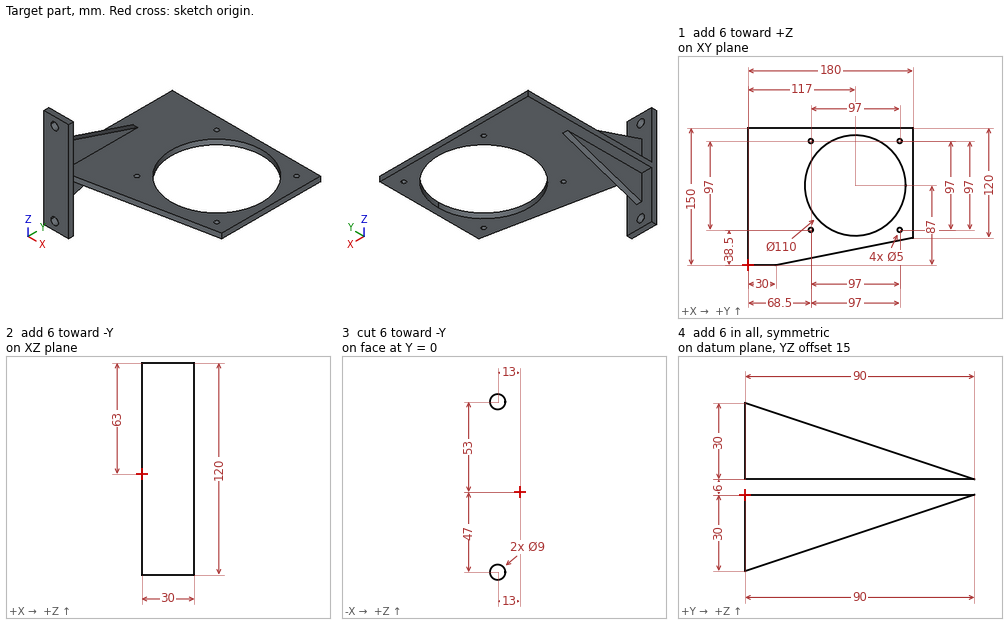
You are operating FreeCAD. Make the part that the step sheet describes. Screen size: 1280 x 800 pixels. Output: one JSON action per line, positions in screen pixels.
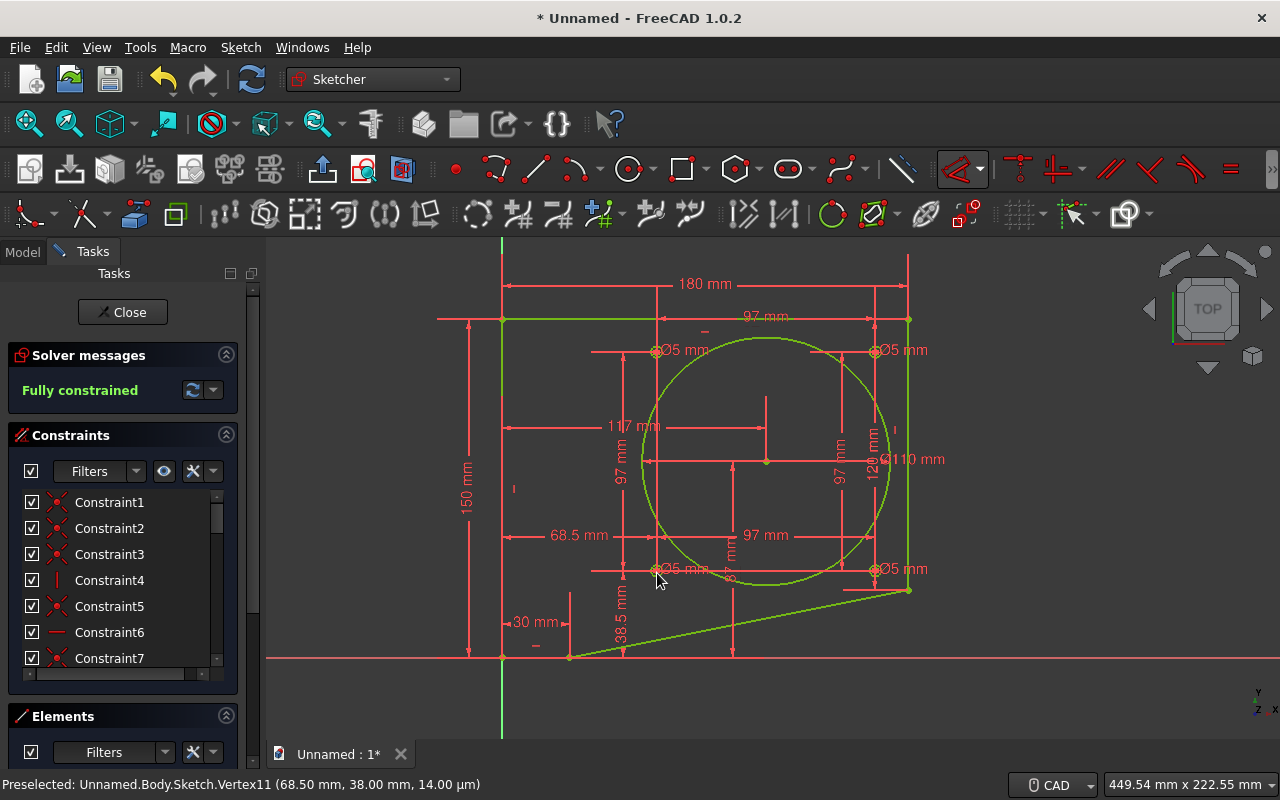
{"action": "left_click", "coordinate": [123, 312]}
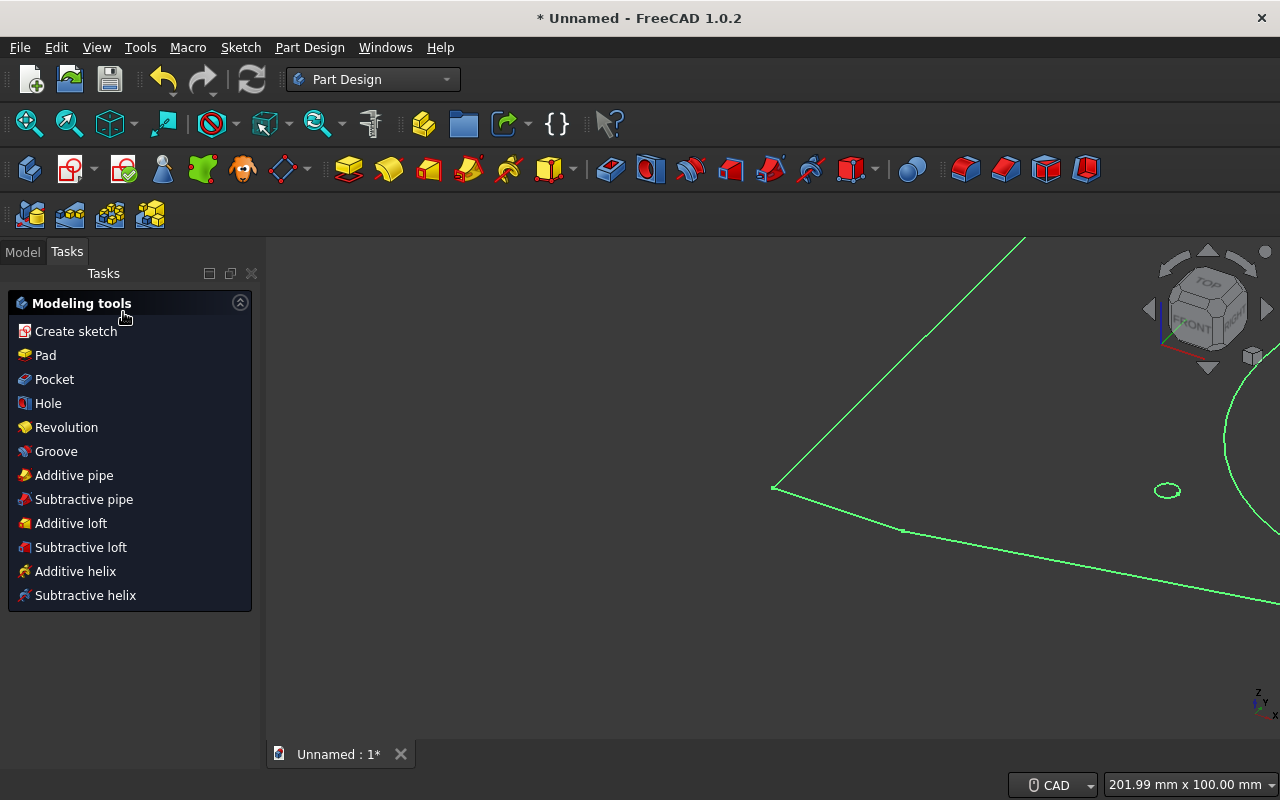
{"action": "left_click", "coordinate": [350, 170]}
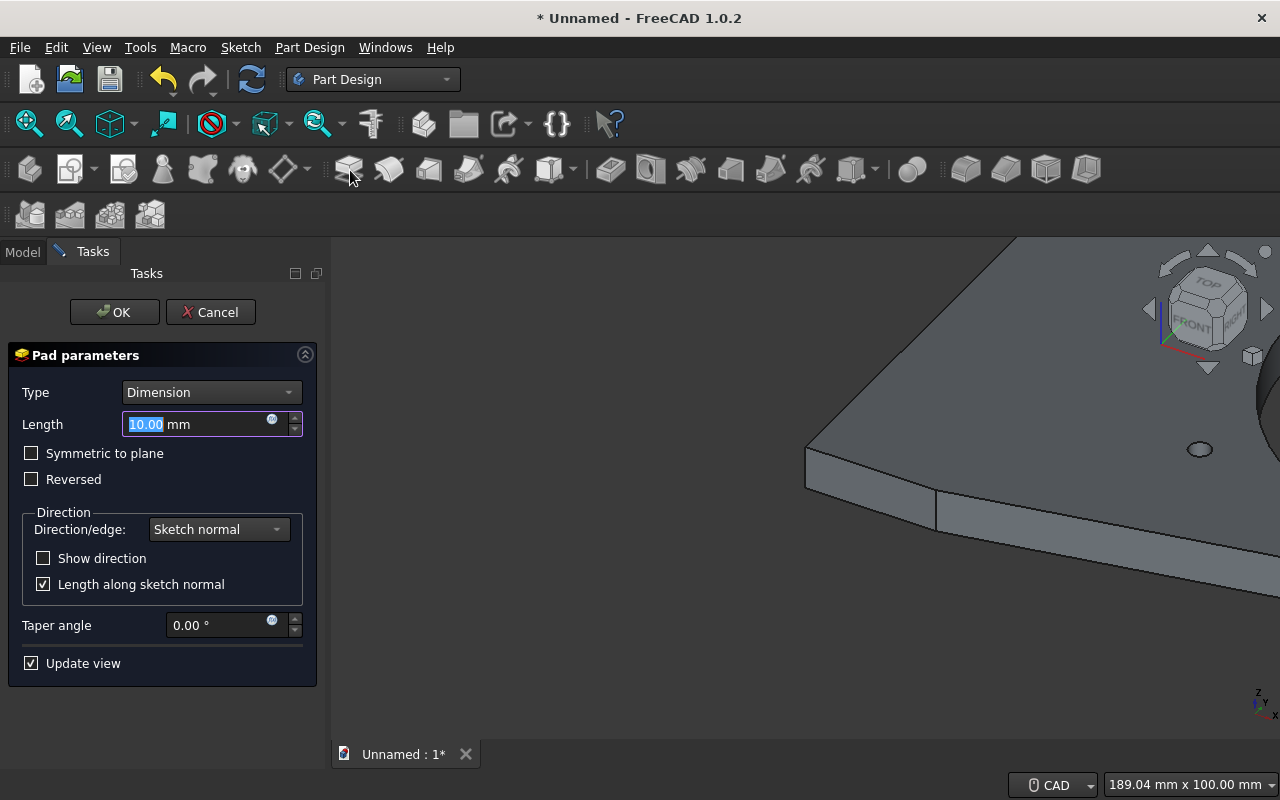
{"action": "type", "text": "6"}
{"action": "key", "text": "Tab"}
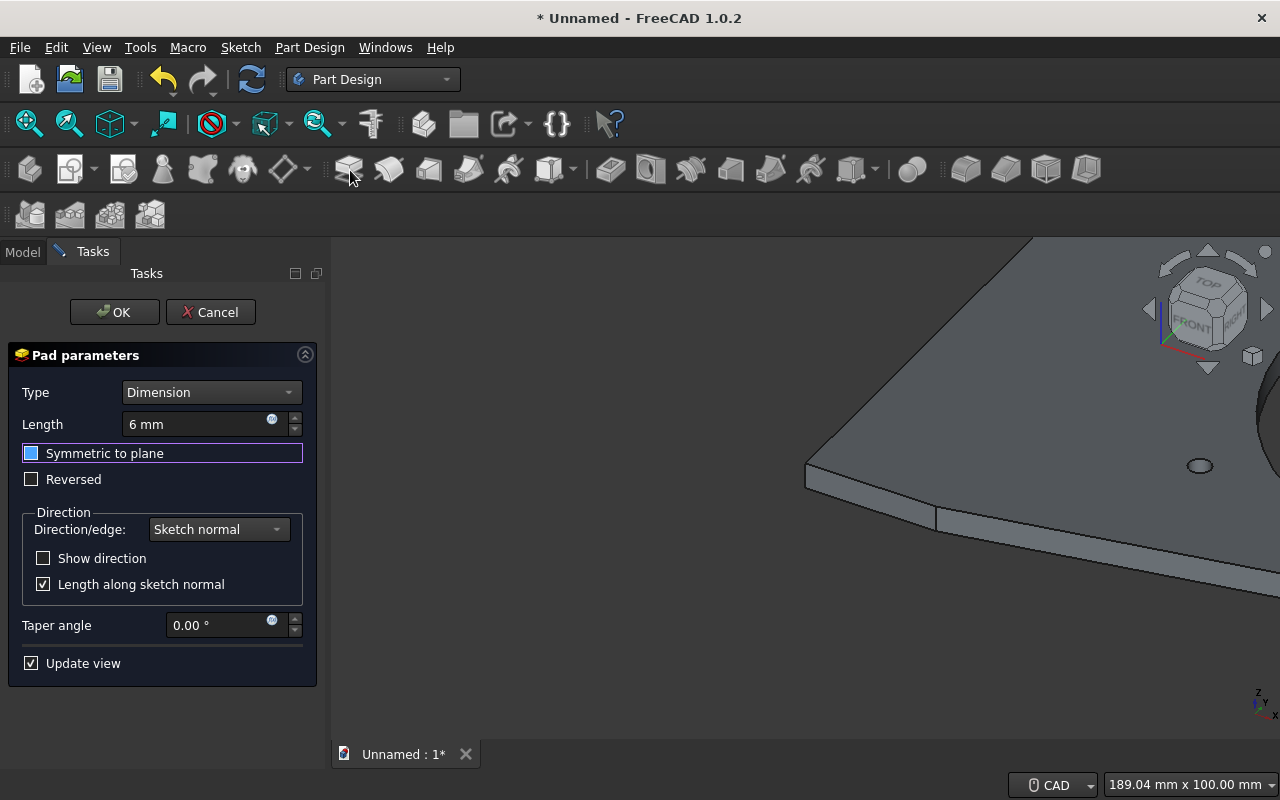
{"action": "left_click", "coordinate": [115, 312]}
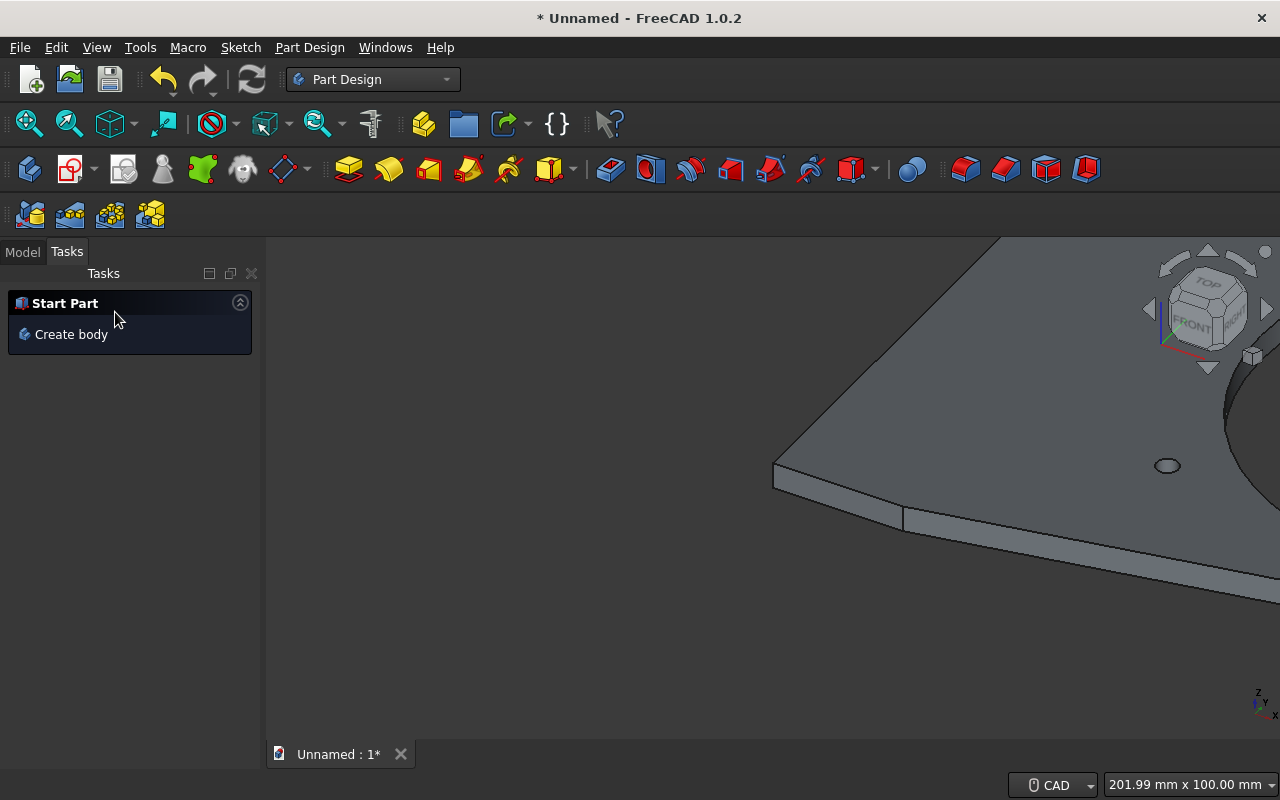
{"action": "key", "text": "v f"}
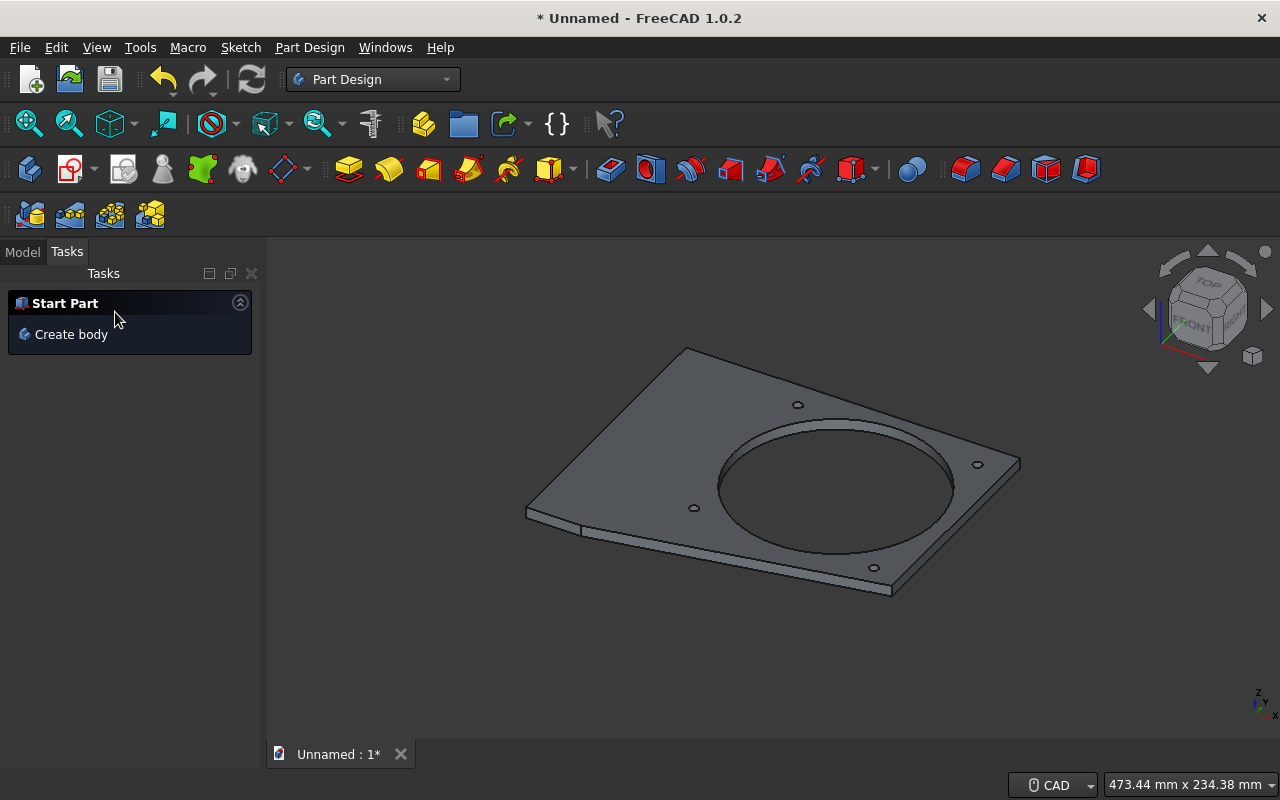
{"action": "left_click", "coordinate": [70, 170]}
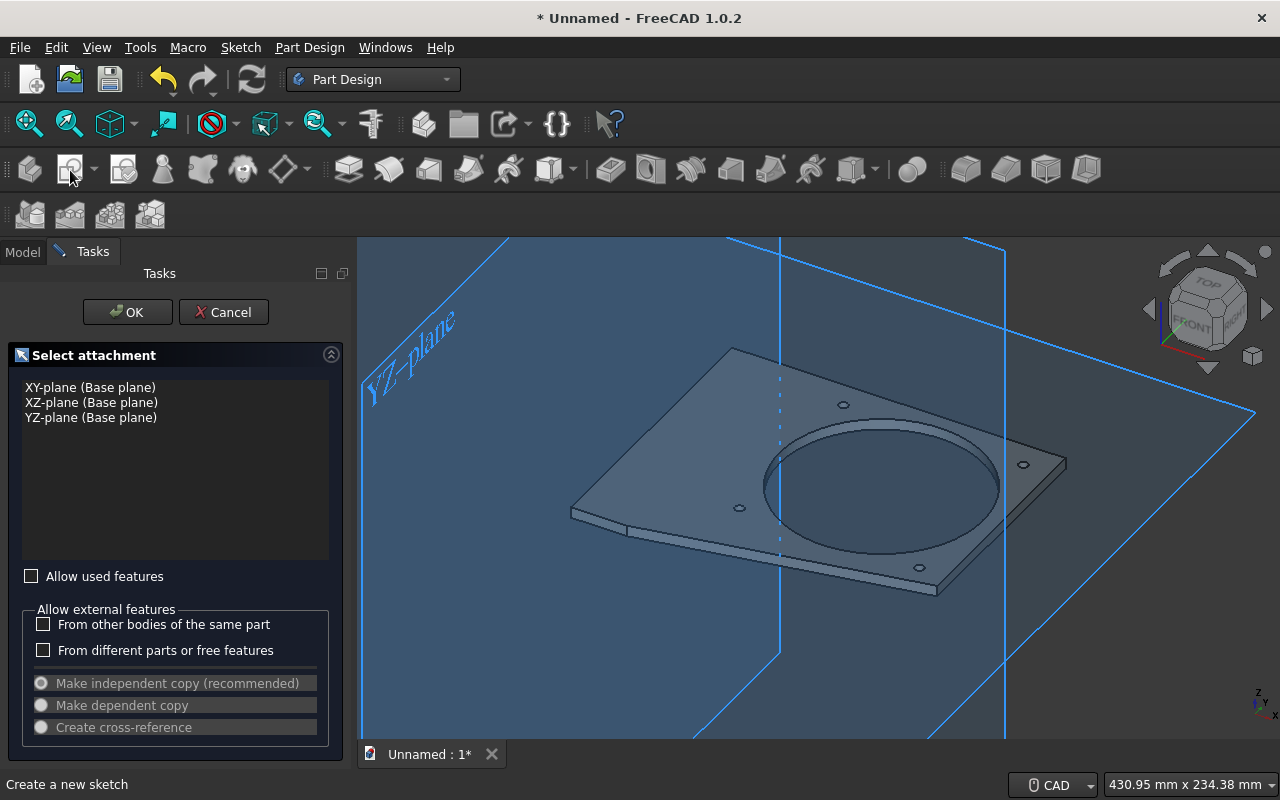
{"action": "left_click", "coordinate": [82, 402]}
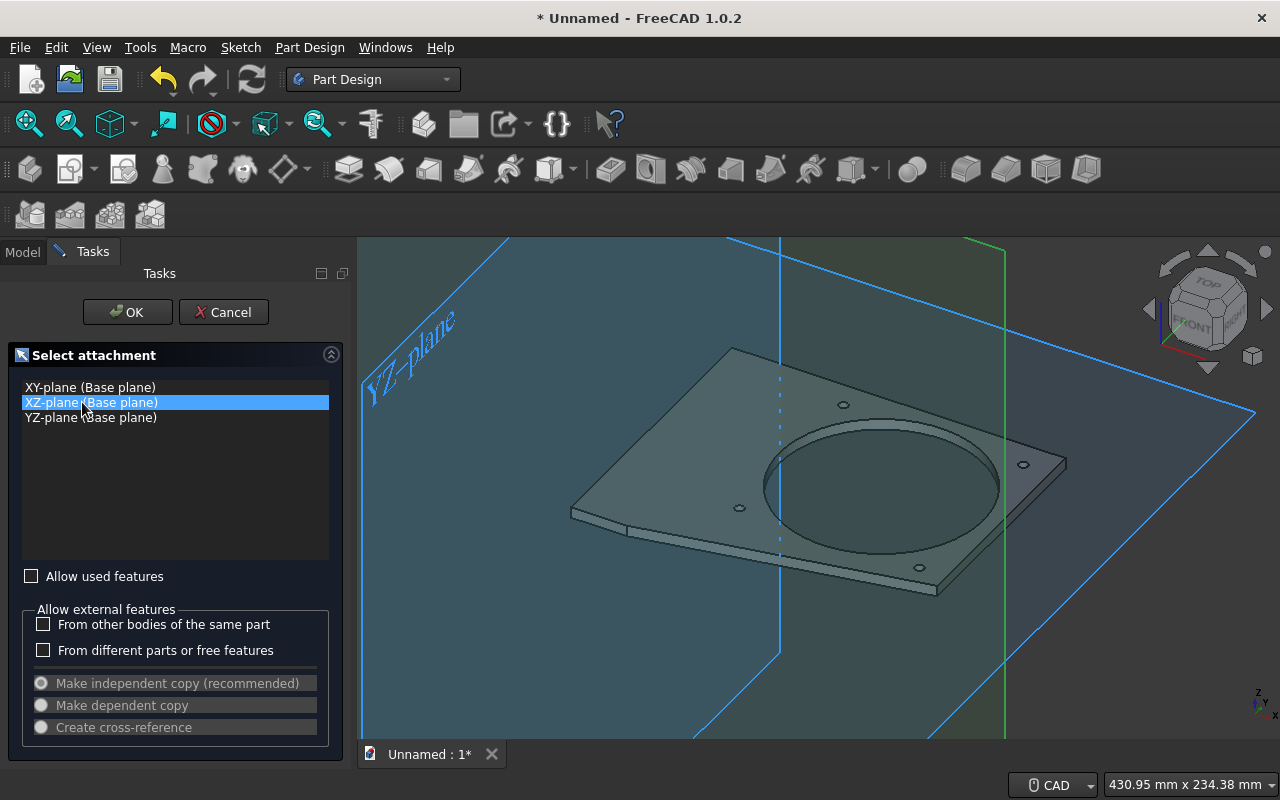
{"action": "left_click", "coordinate": [128, 312]}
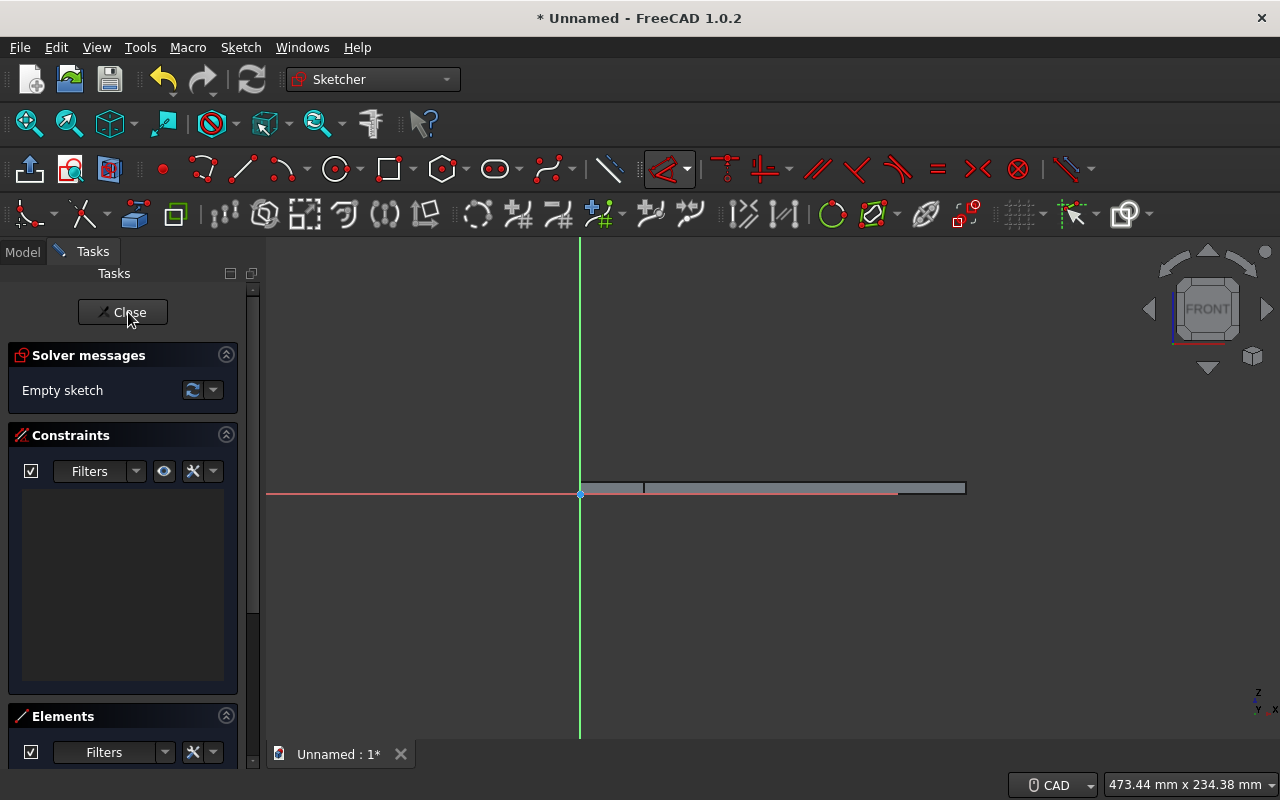
{"action": "key", "text": "g r"}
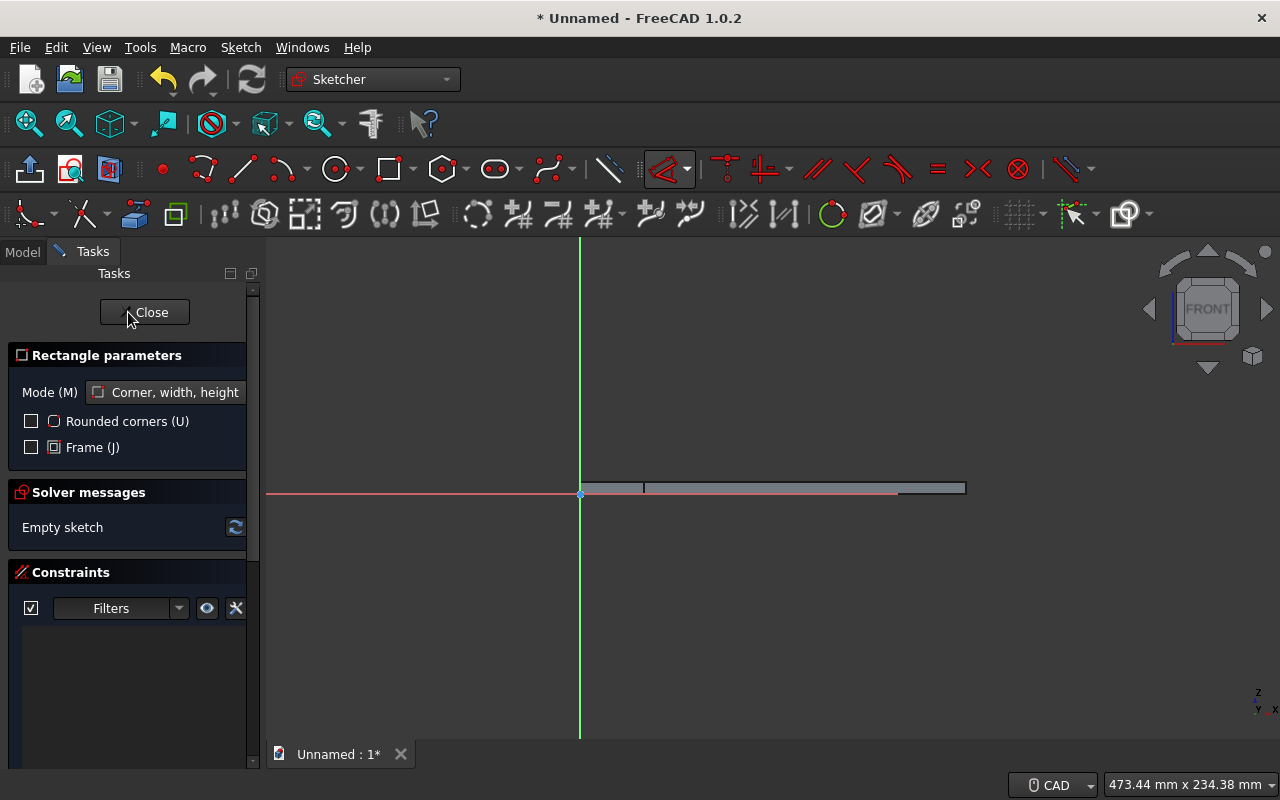
{"action": "left_click", "coordinate": [580, 359]}
{"action": "mouse_move", "coordinate": [644, 617]}